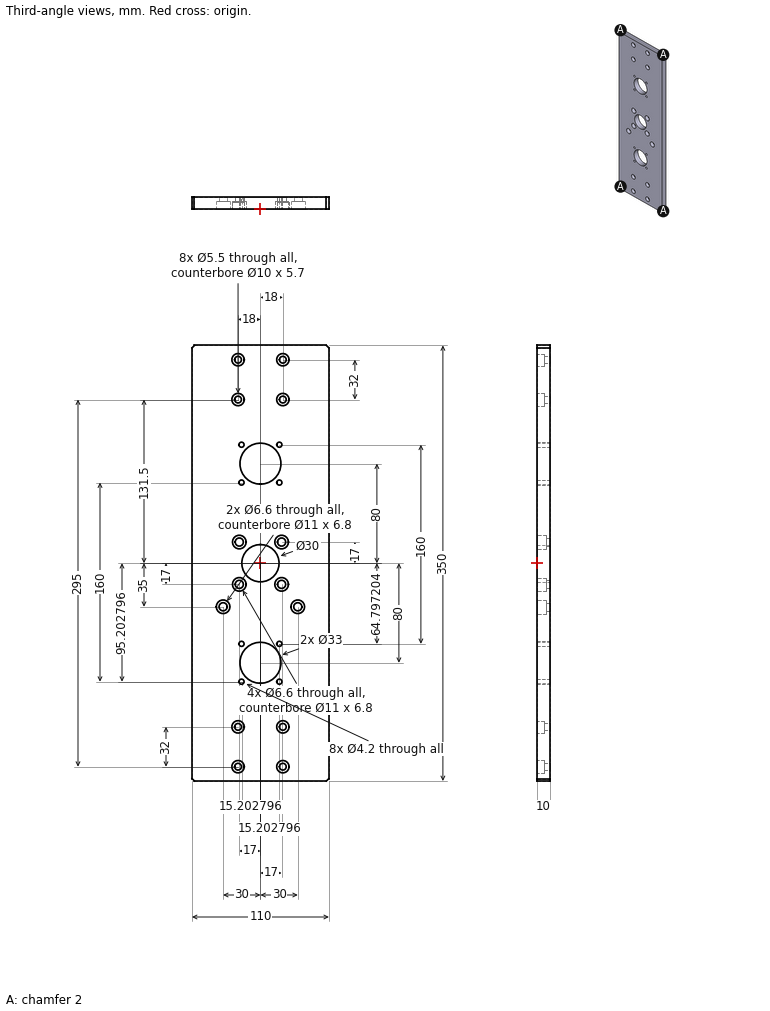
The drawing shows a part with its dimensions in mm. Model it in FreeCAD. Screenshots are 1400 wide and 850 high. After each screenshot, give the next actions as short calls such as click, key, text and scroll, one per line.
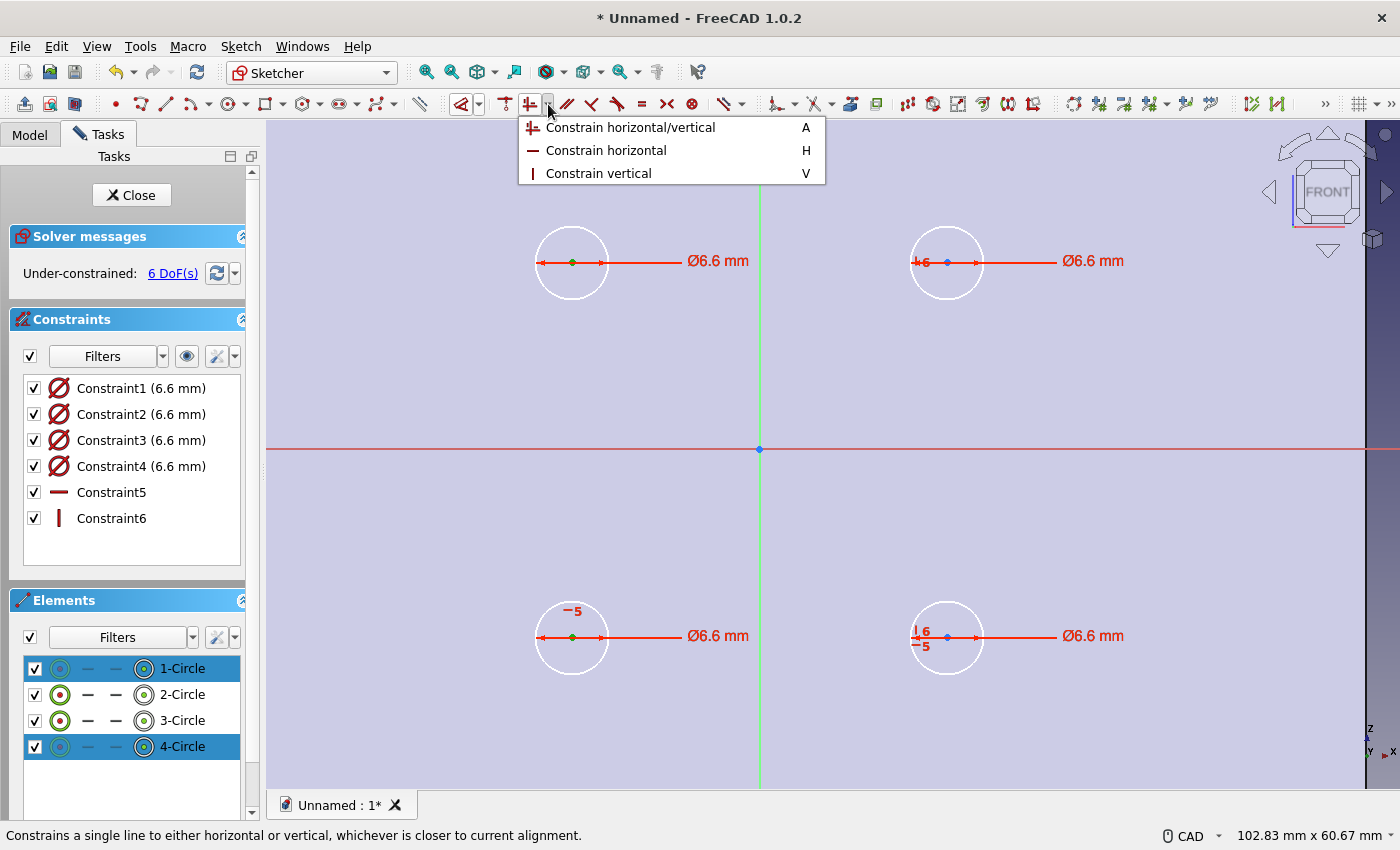
click(672, 174)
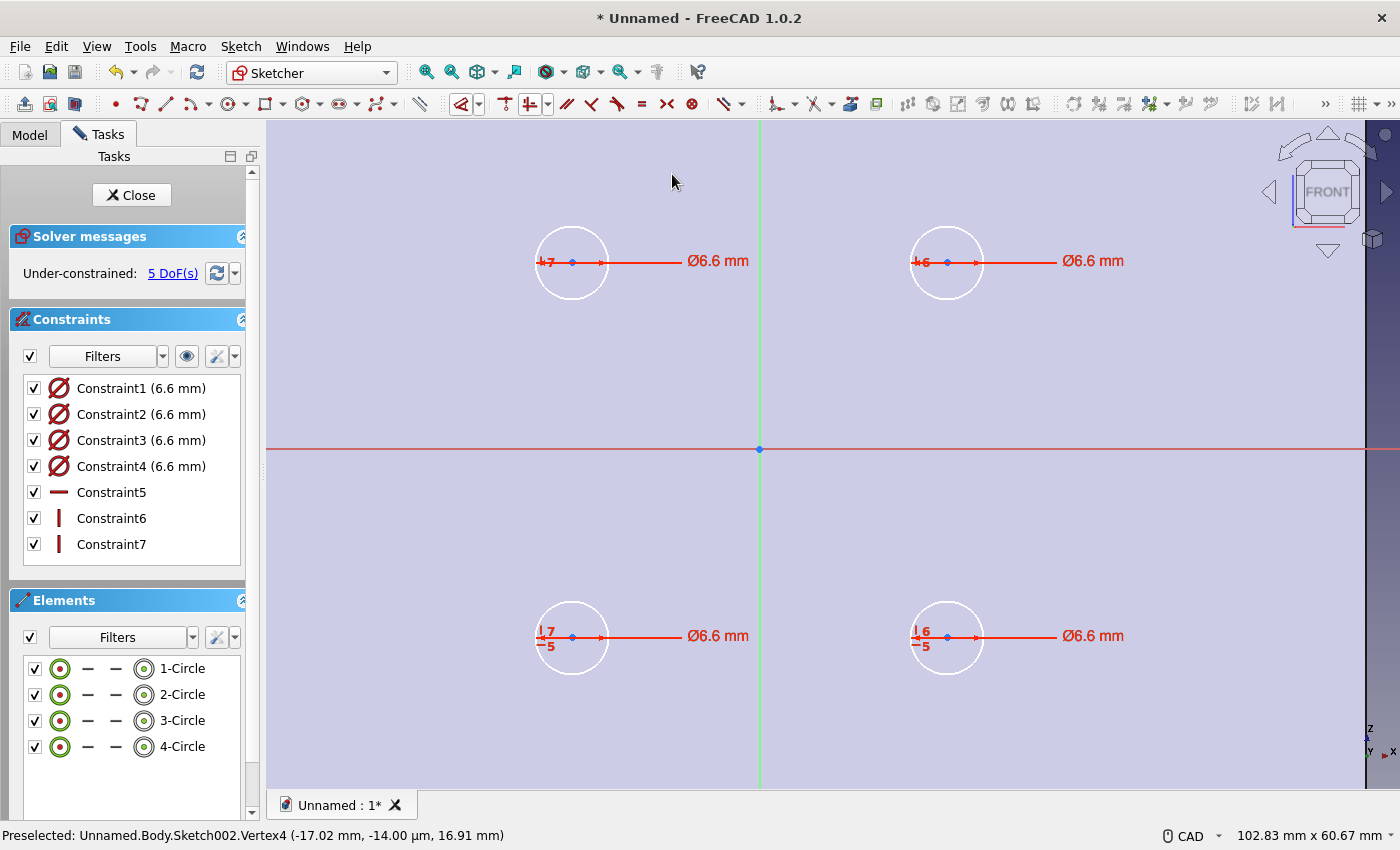
click(947, 263)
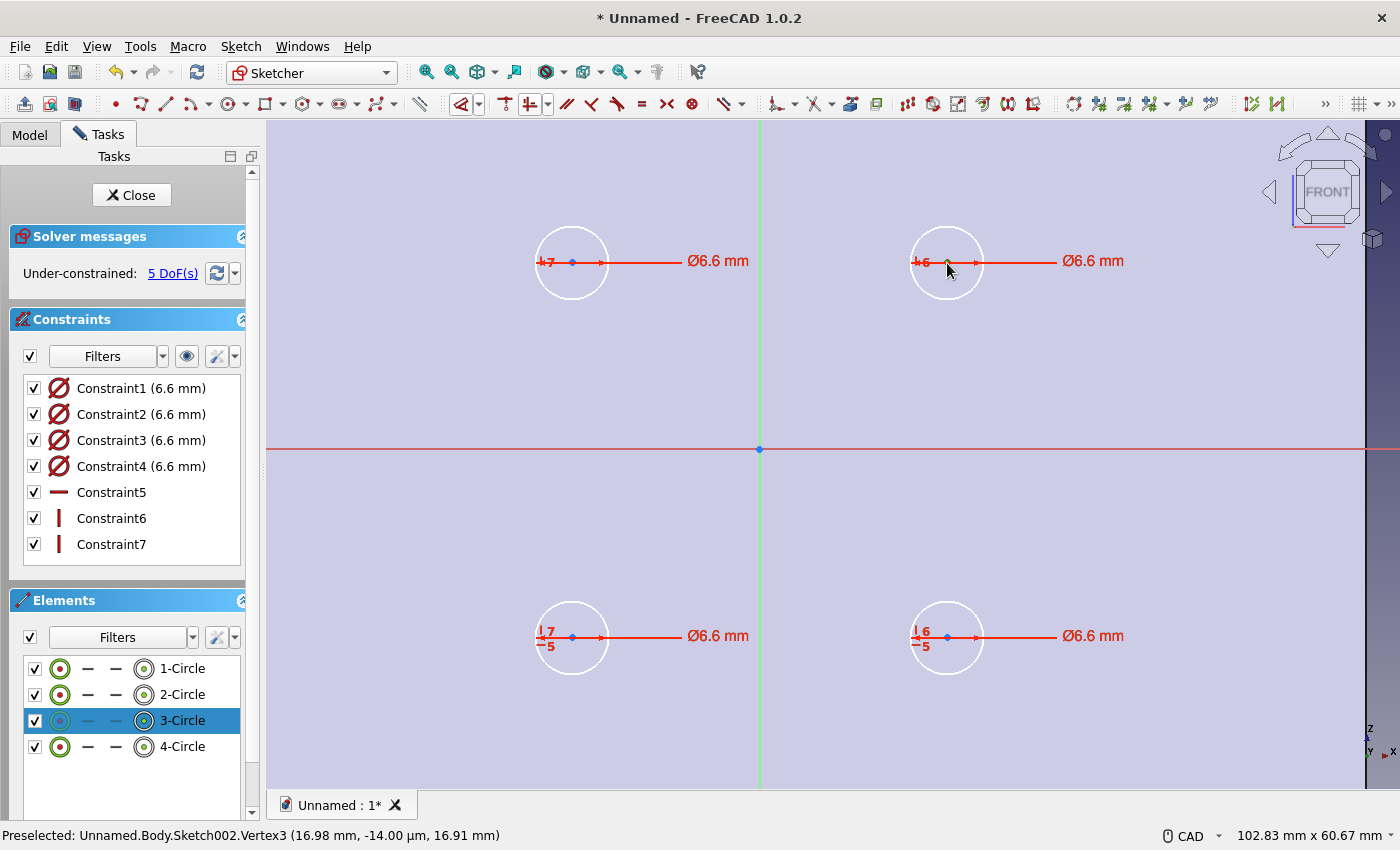
click(572, 263)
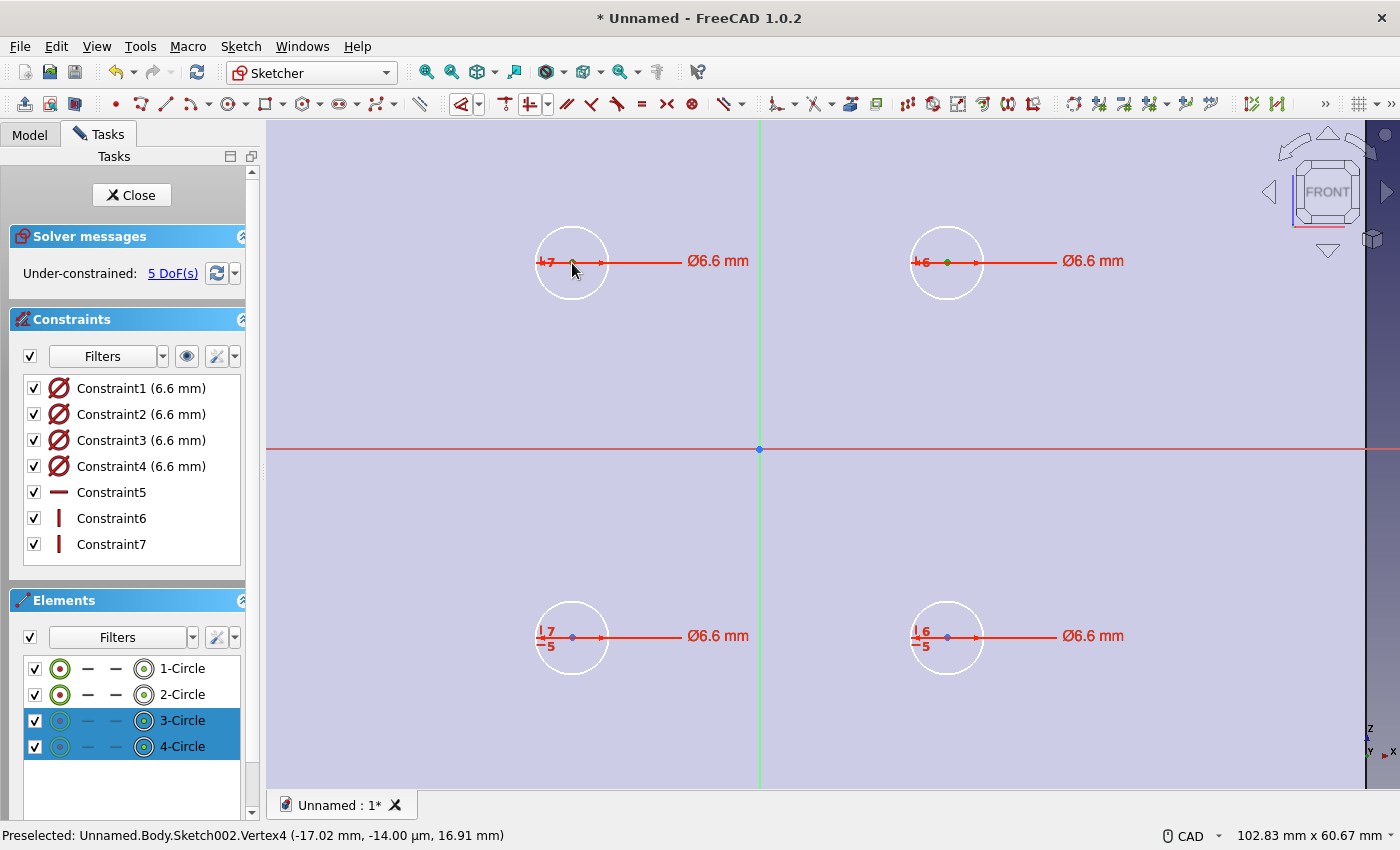
key(h)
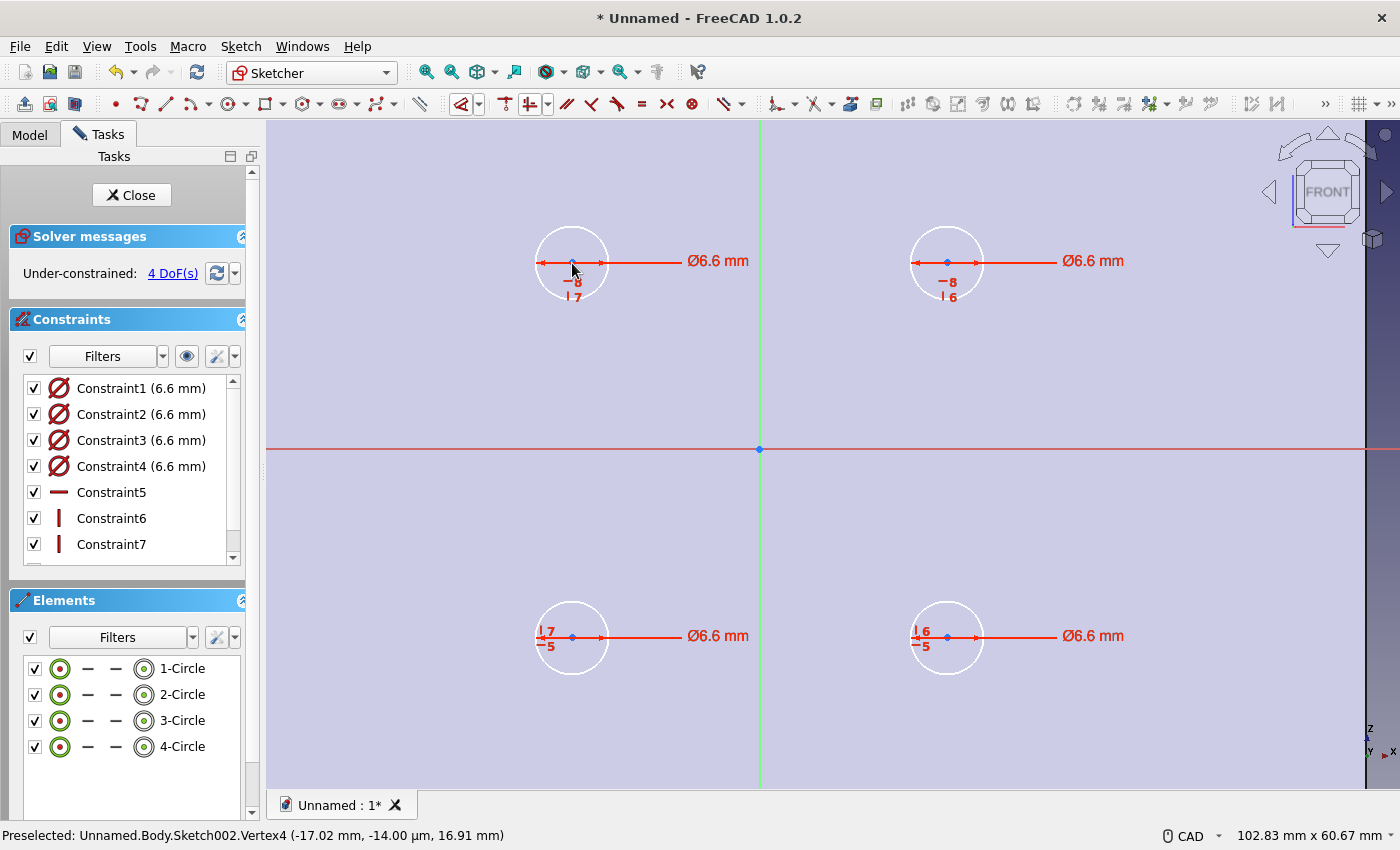
click(572, 638)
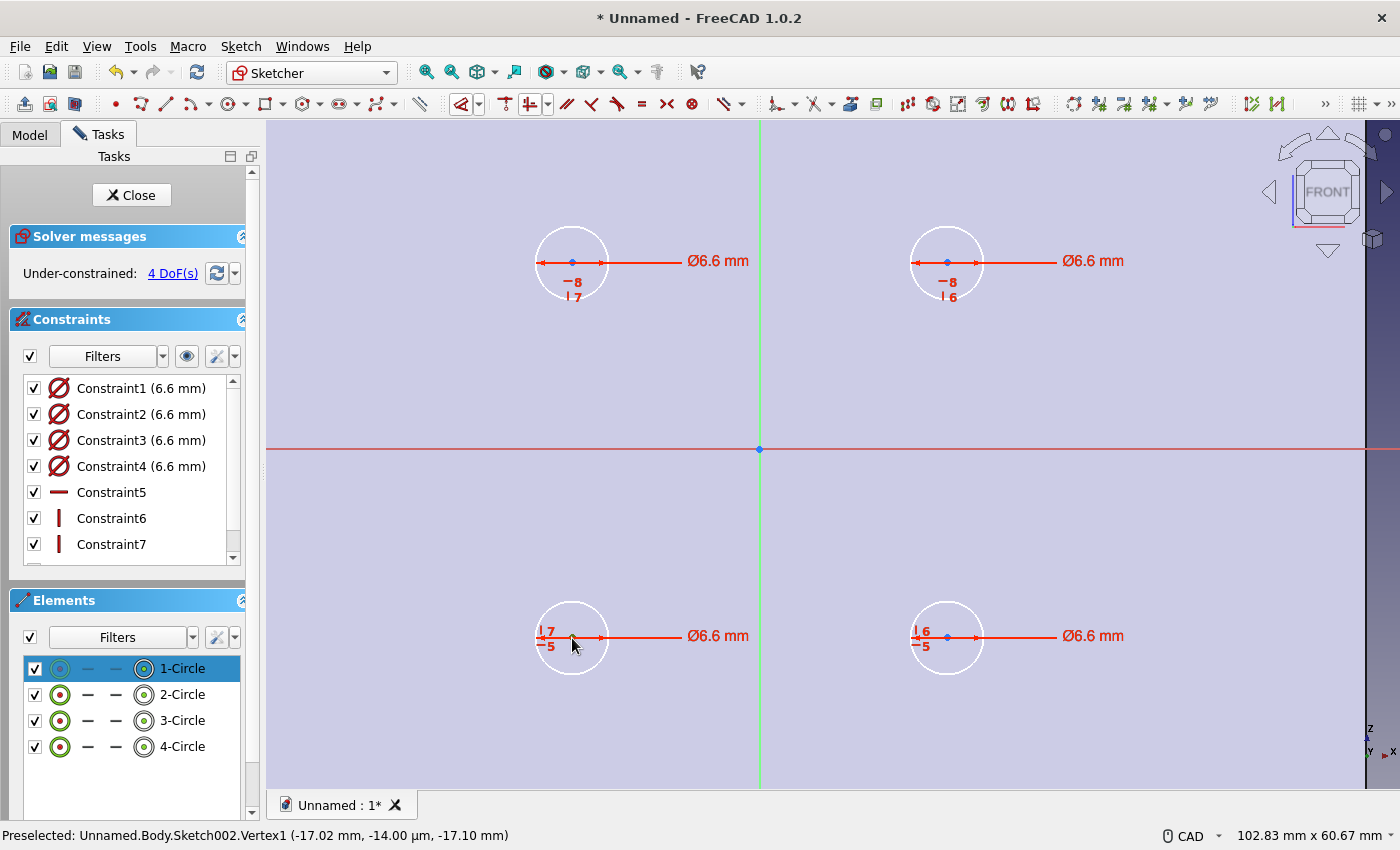
key(l)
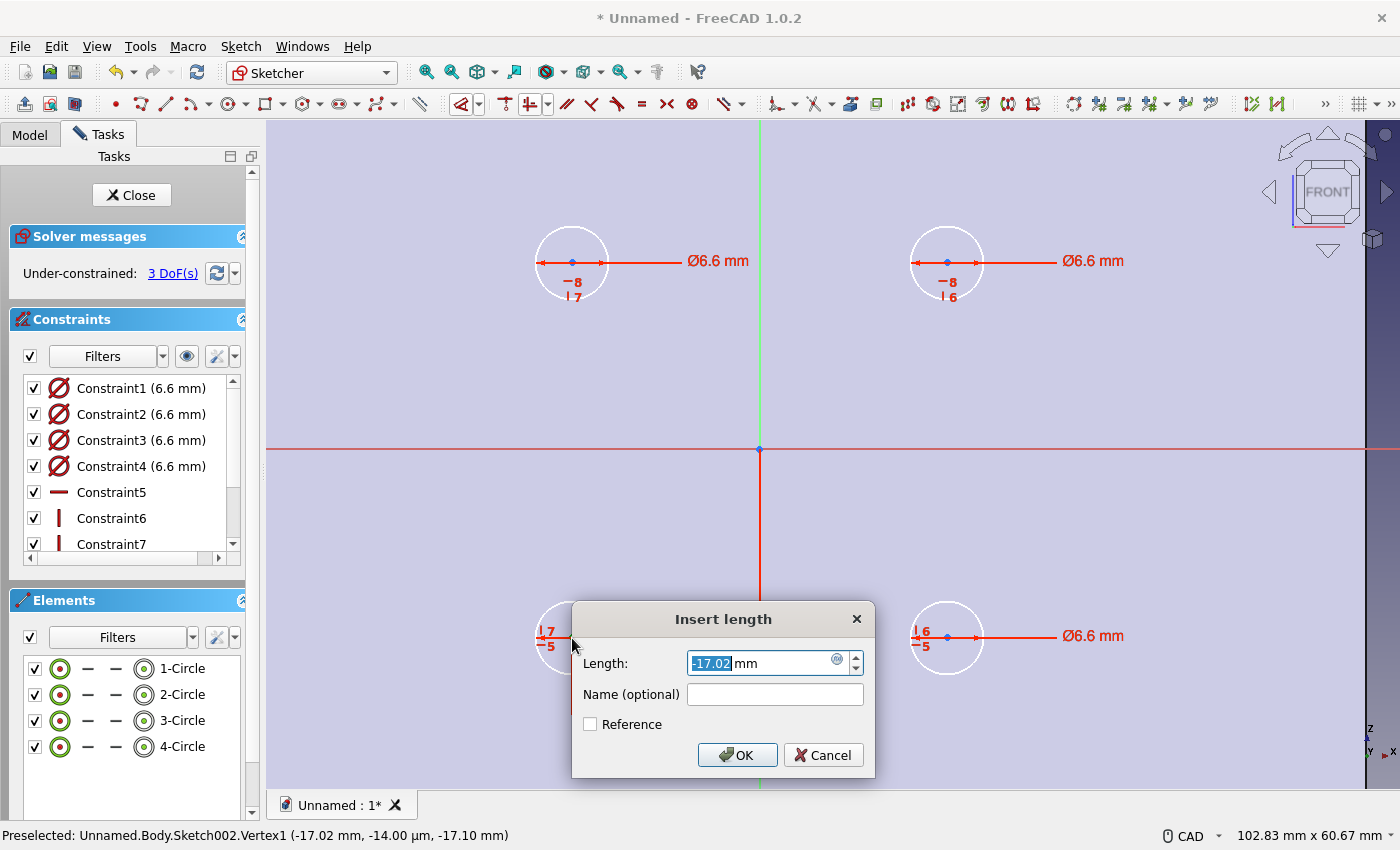
text(-17)
key(Return)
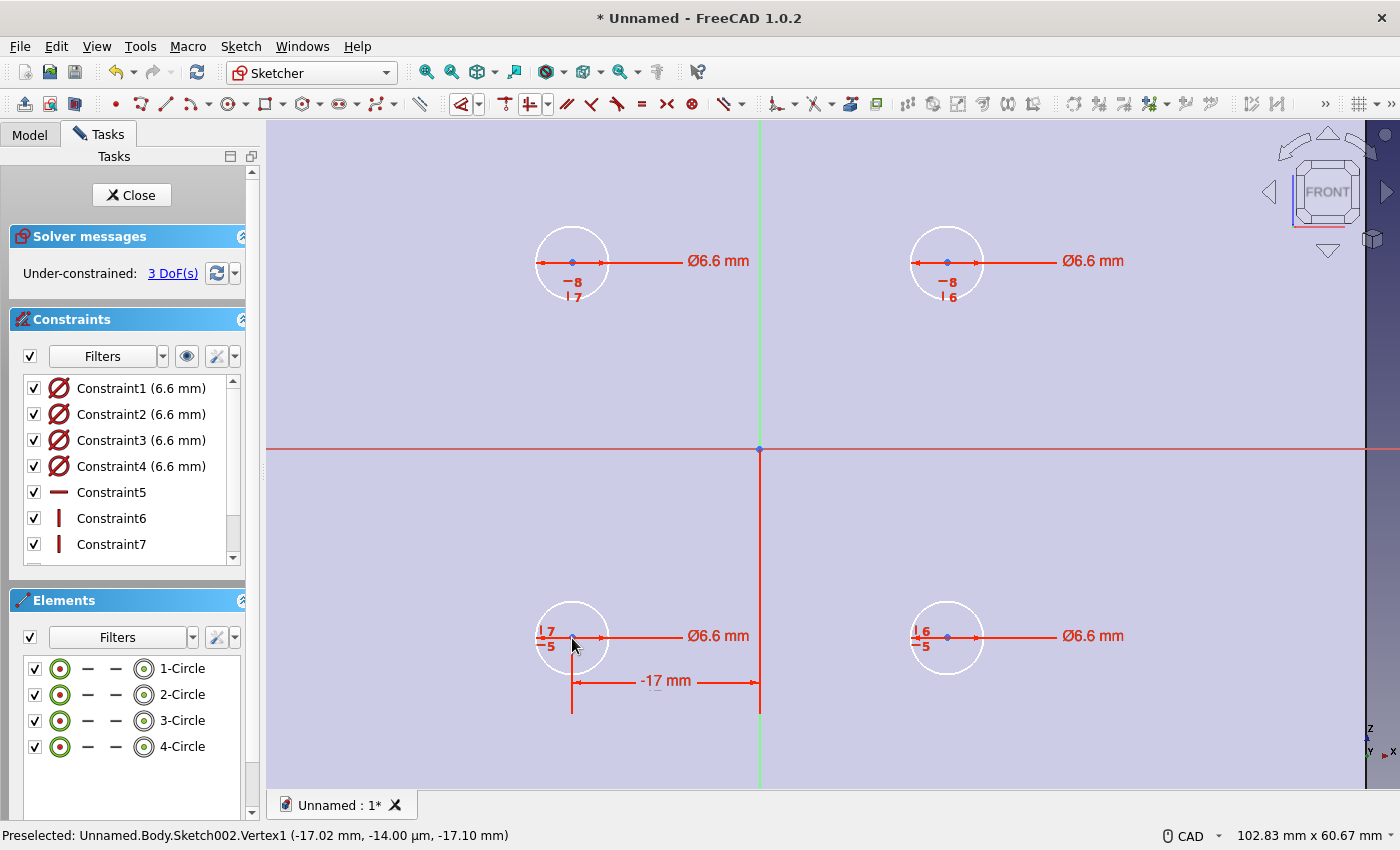
click(572, 638)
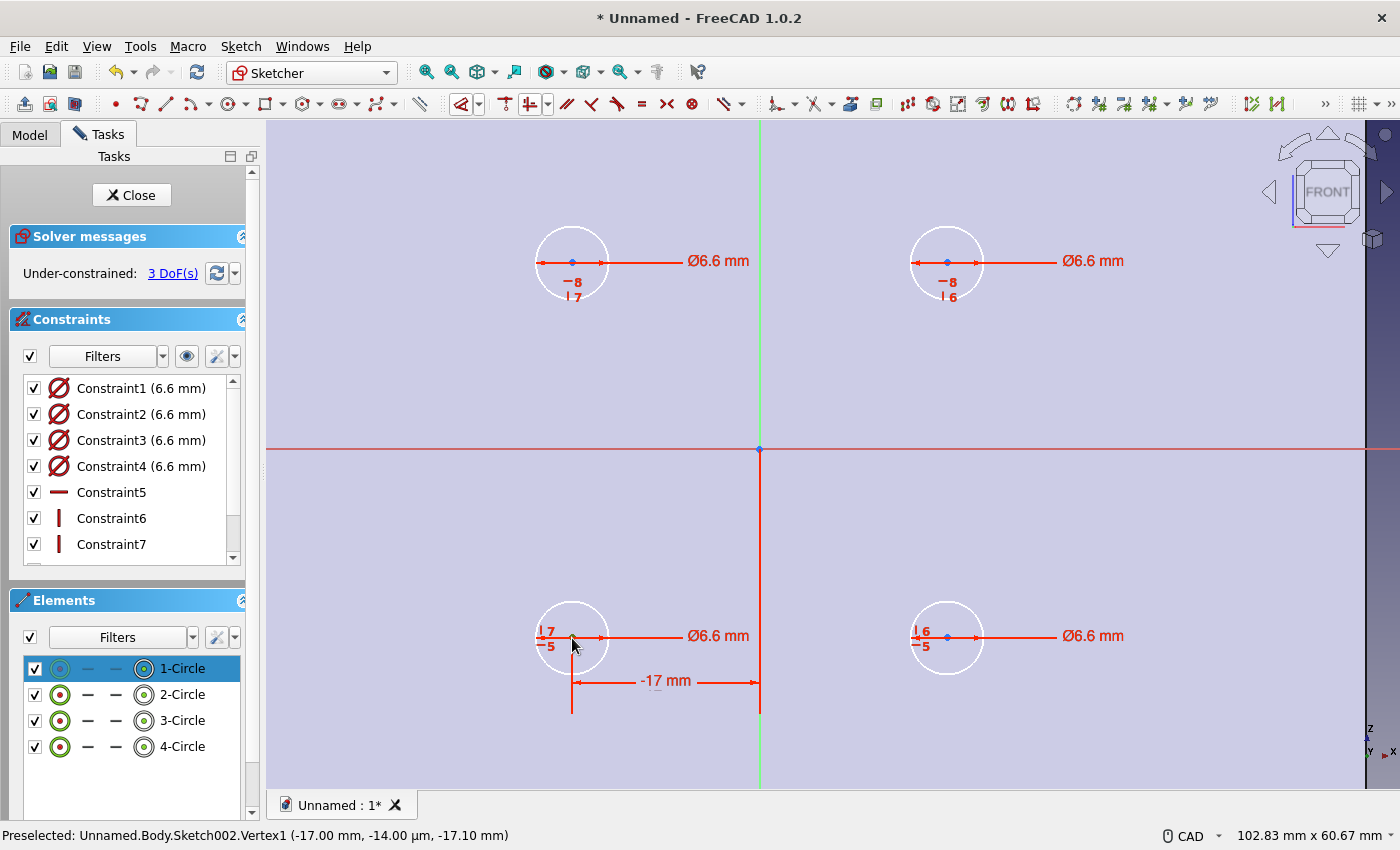
click(478, 104)